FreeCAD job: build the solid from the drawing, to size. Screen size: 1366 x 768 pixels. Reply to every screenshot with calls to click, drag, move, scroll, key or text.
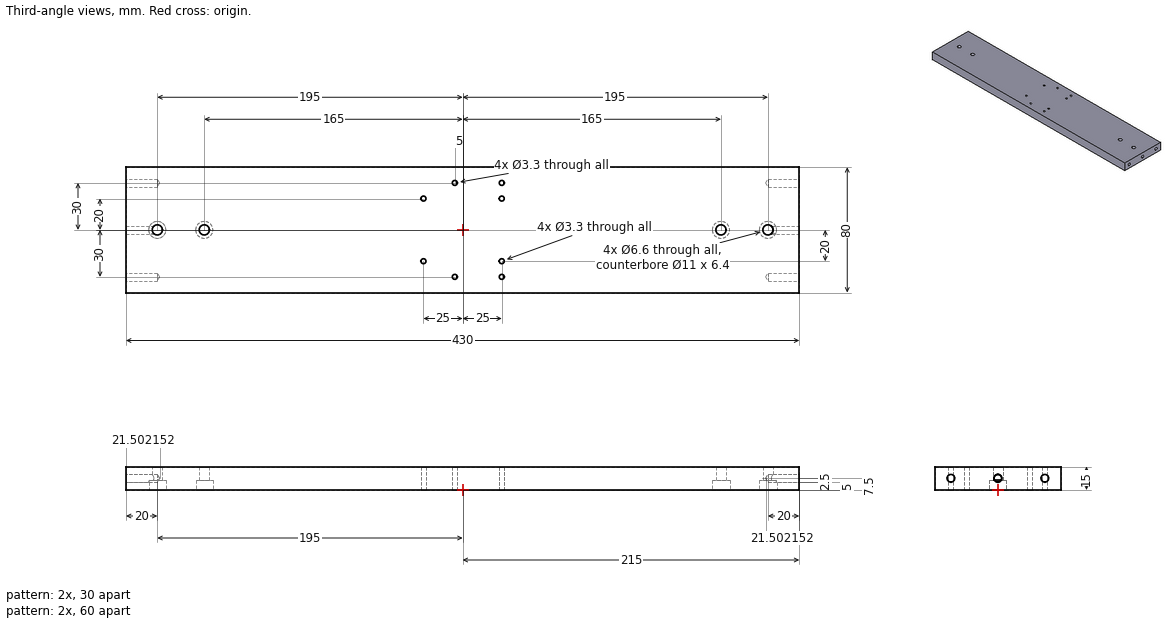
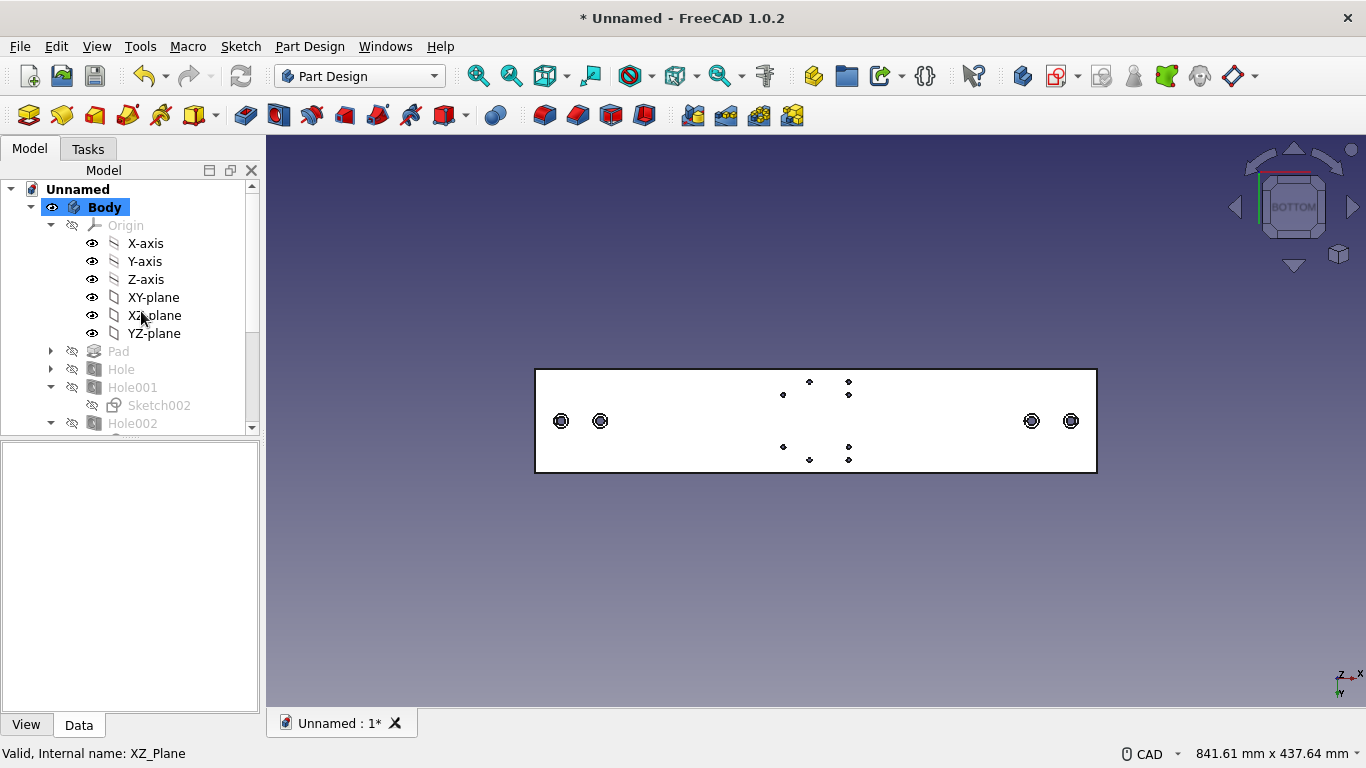
click(137, 315)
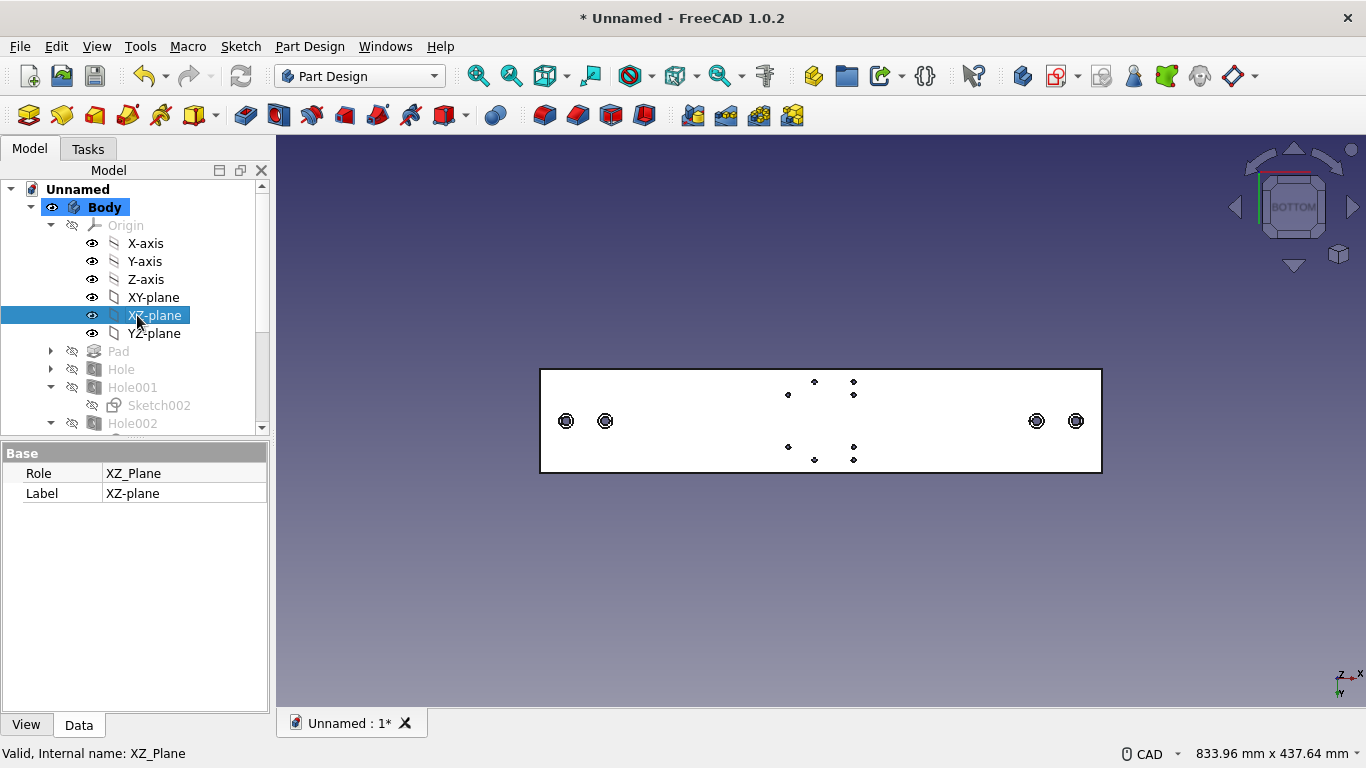
click(1232, 76)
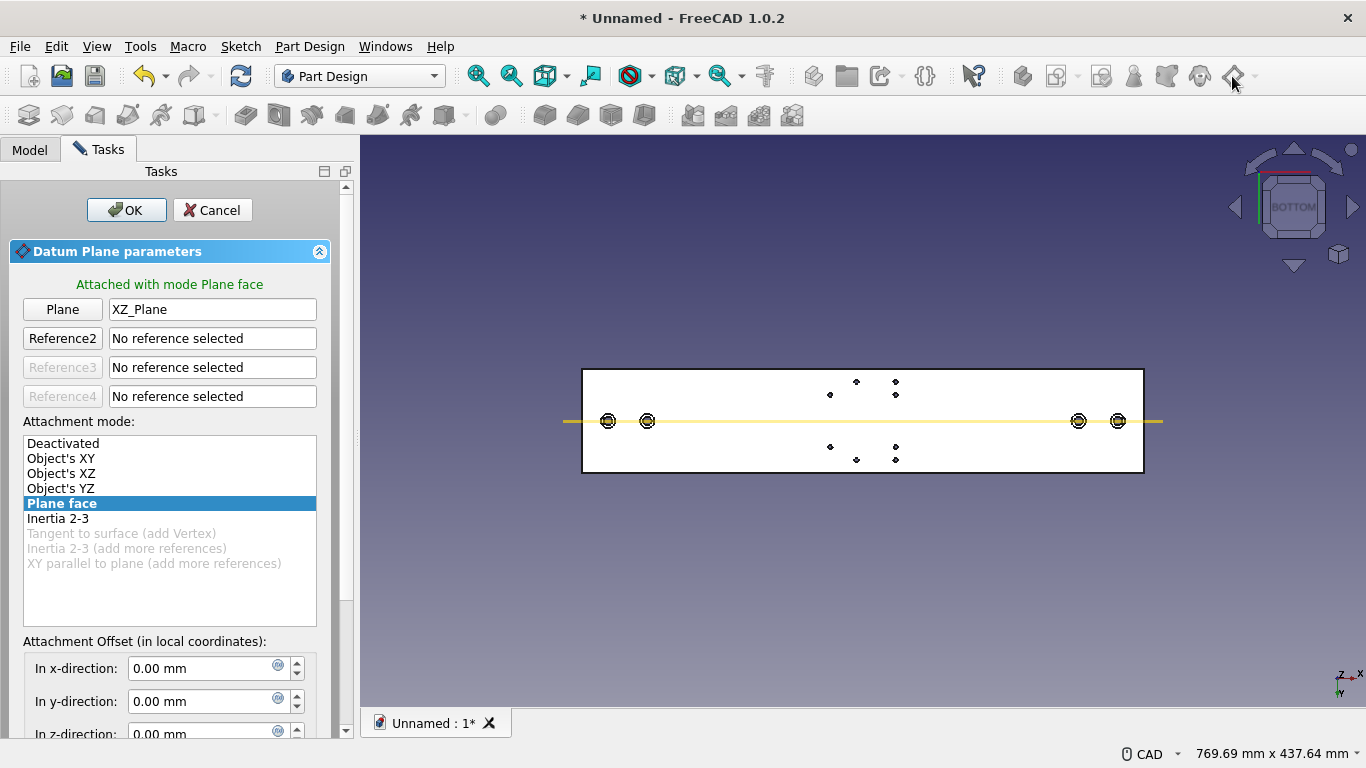
scroll(346, 460, down, 2)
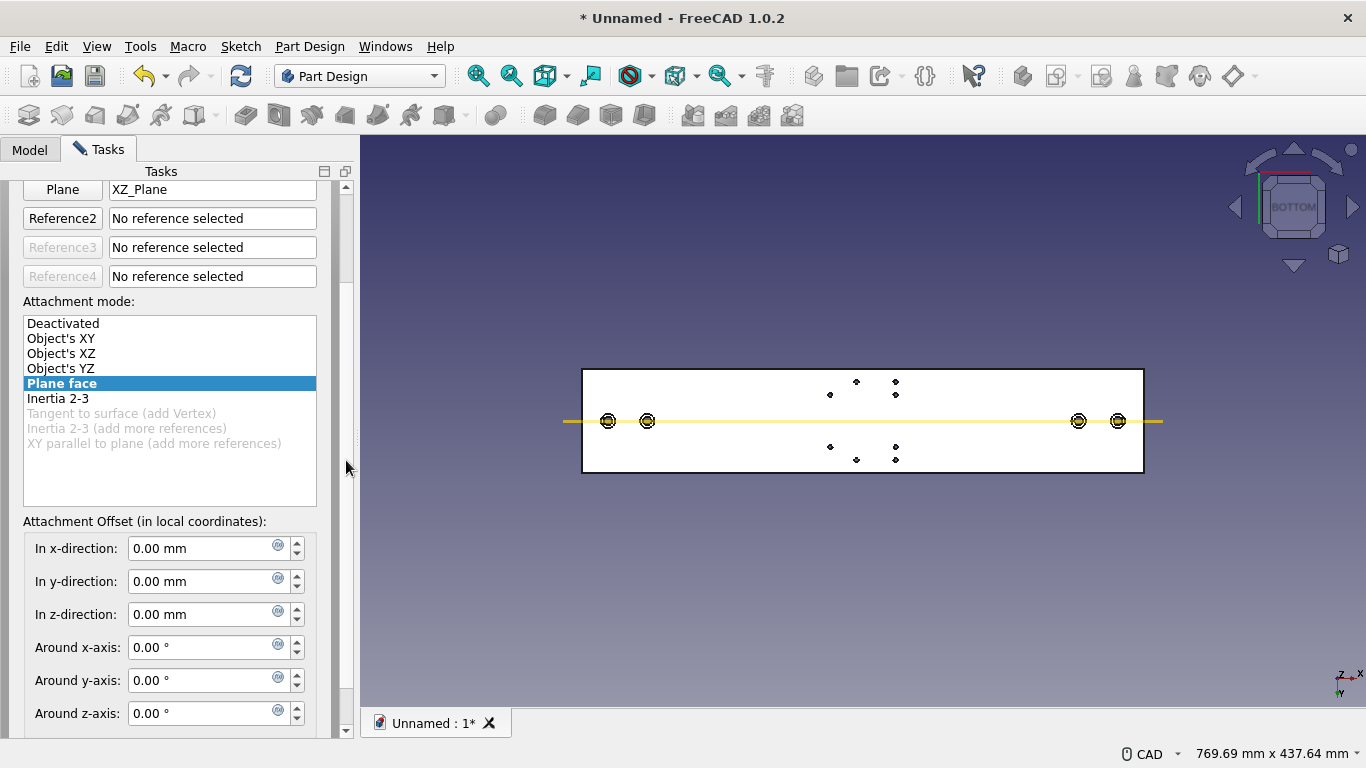
triple_click(210, 614)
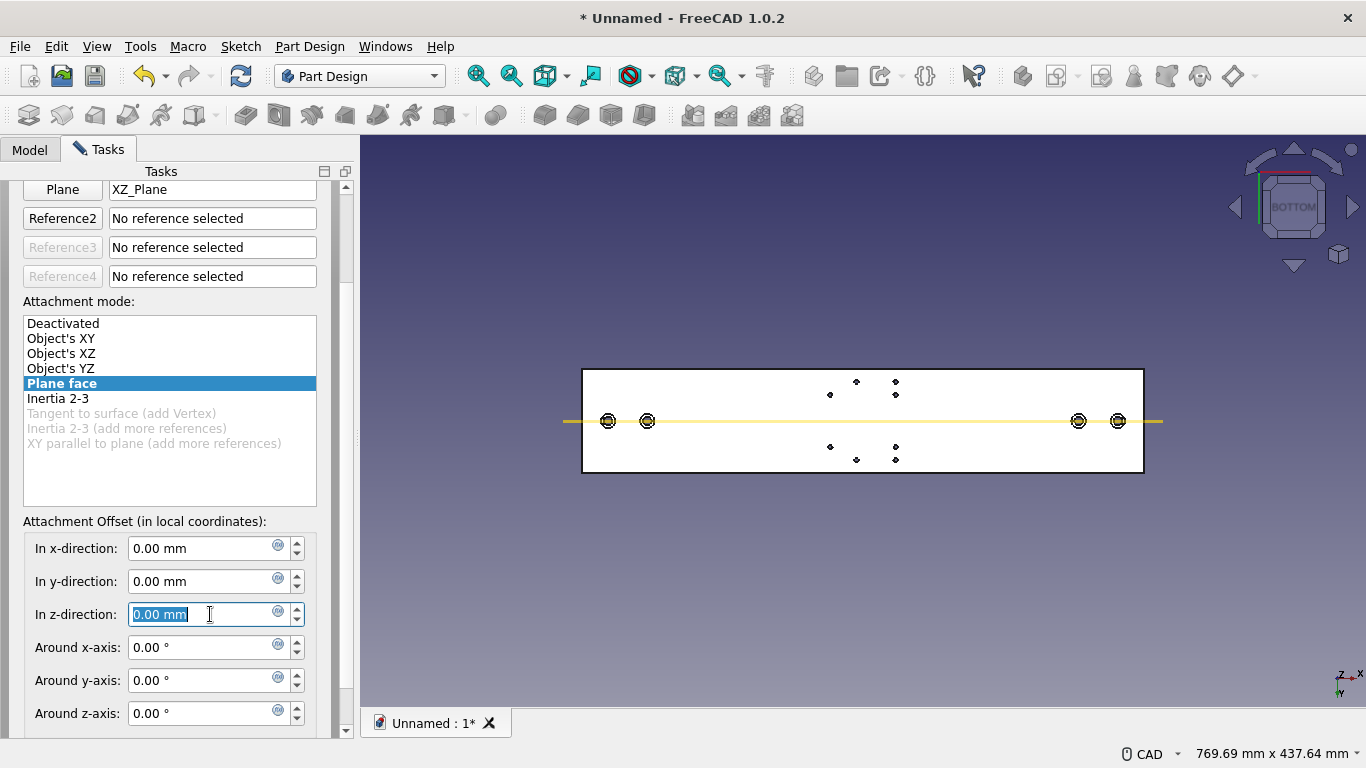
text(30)
key(Tab)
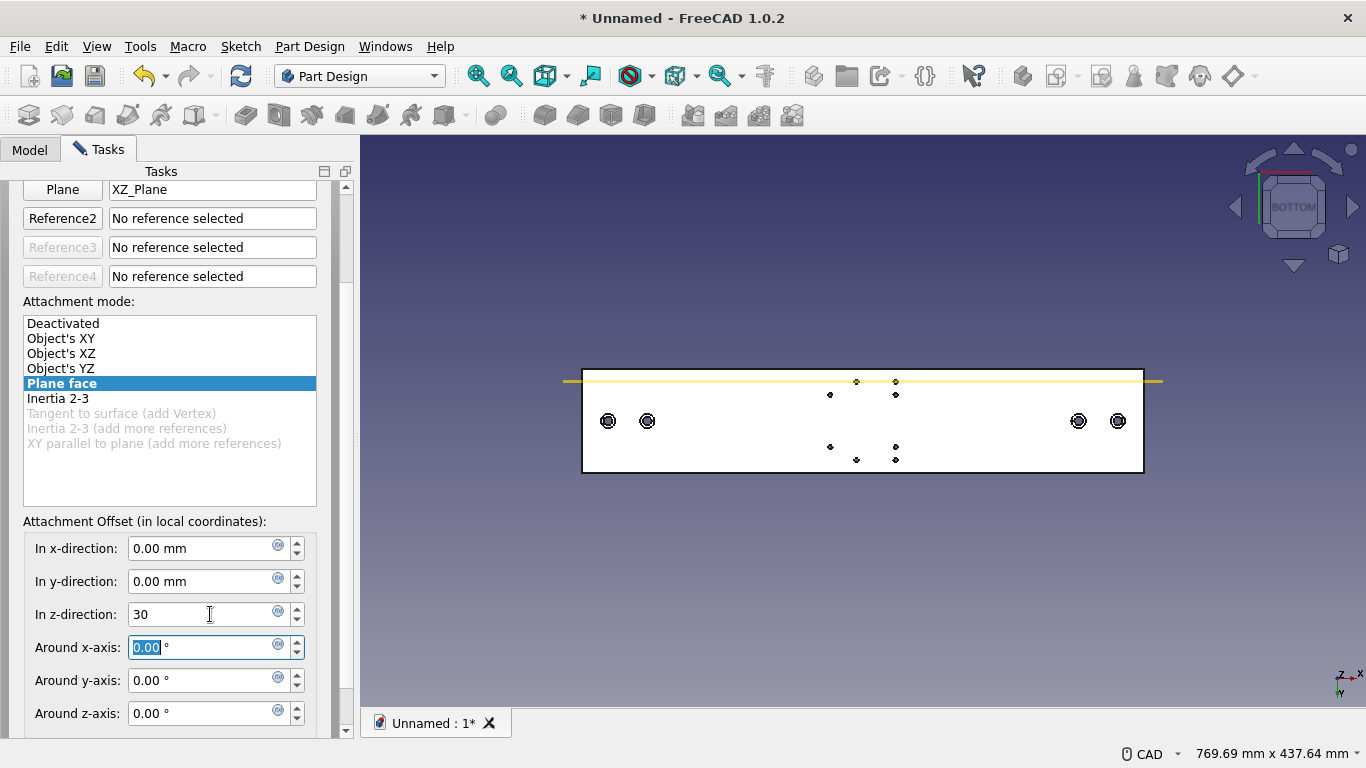
scroll(346, 460, up, 3)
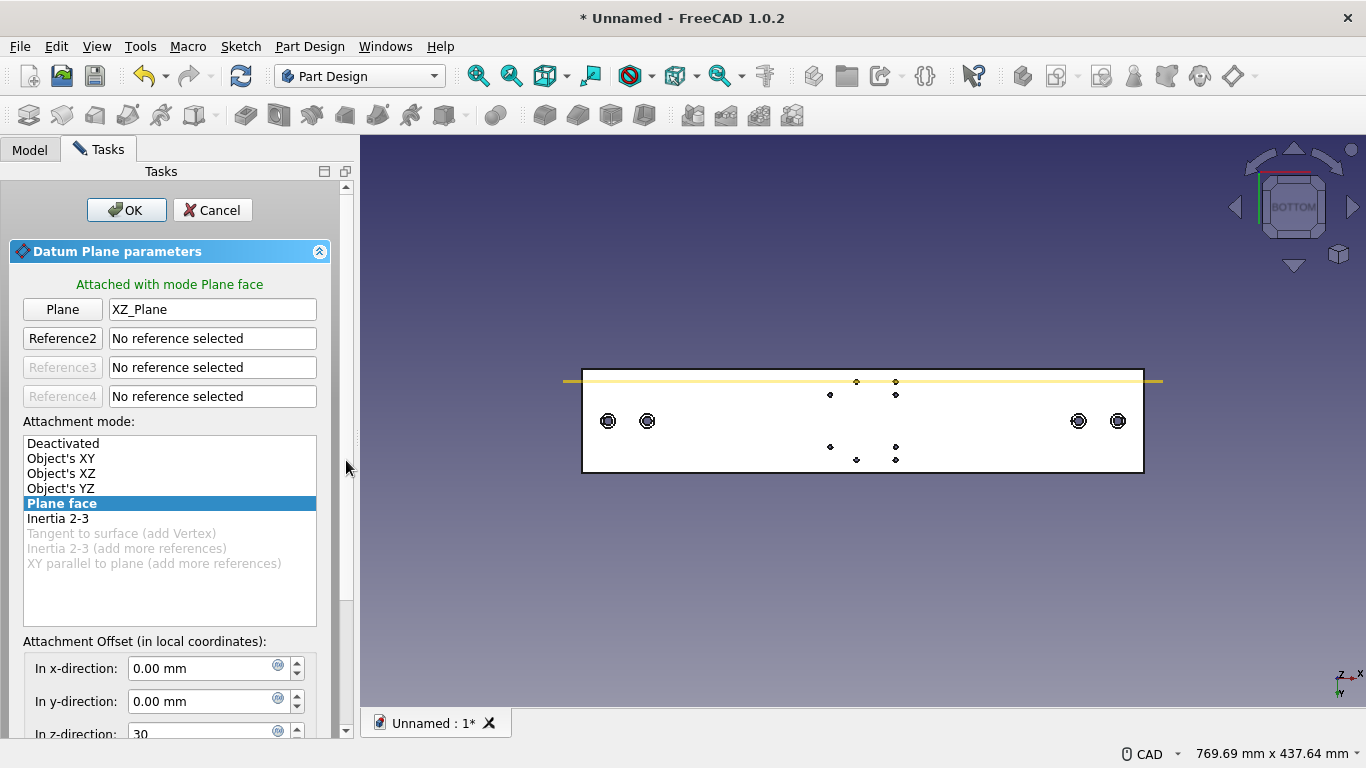
click(127, 210)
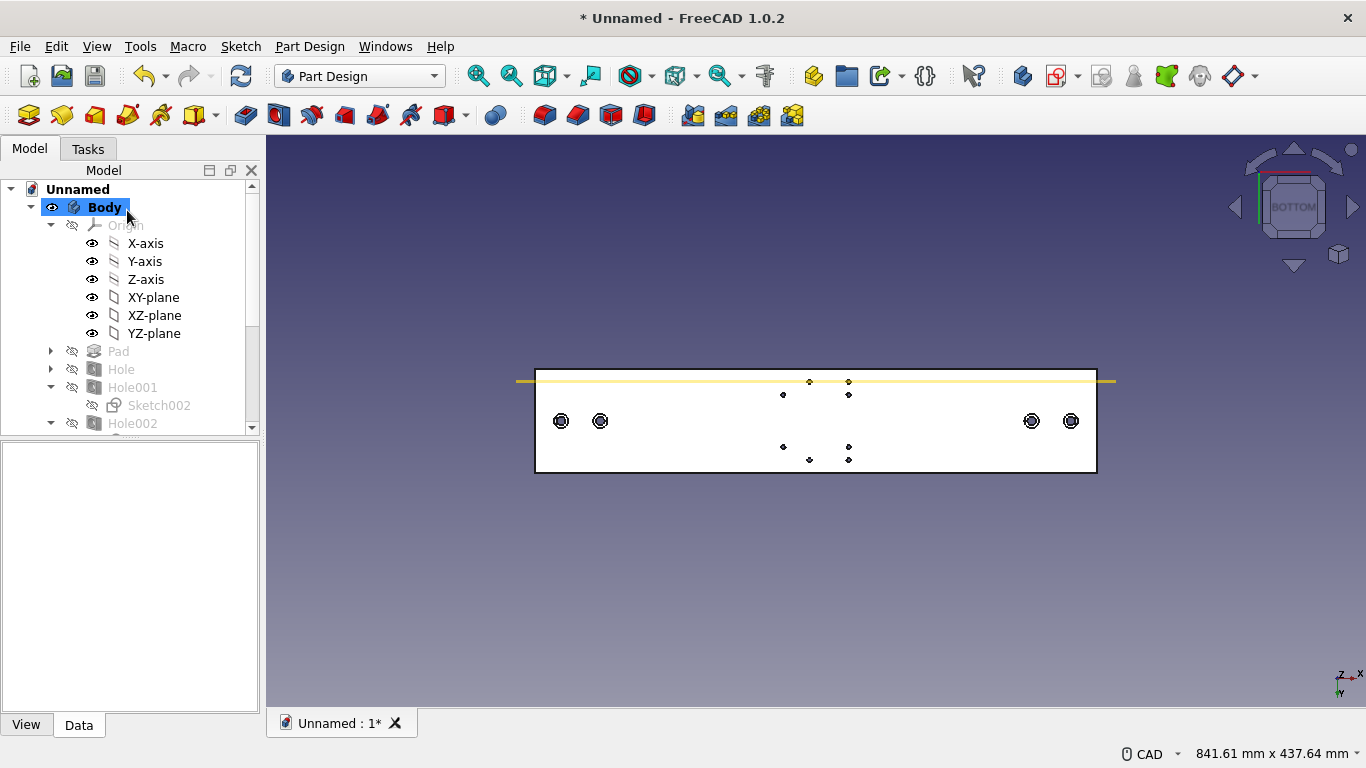
scroll(101, 311, down, 3)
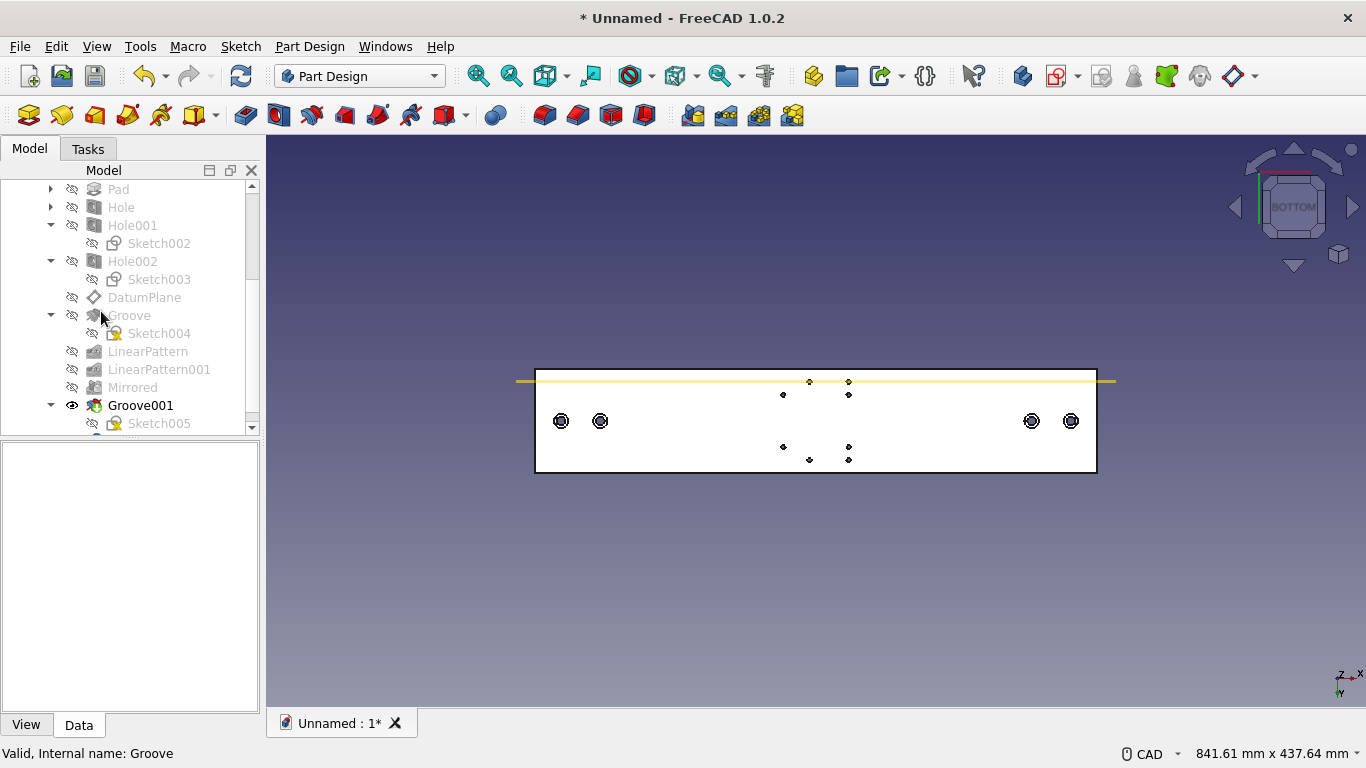
scroll(141, 311, up, 15)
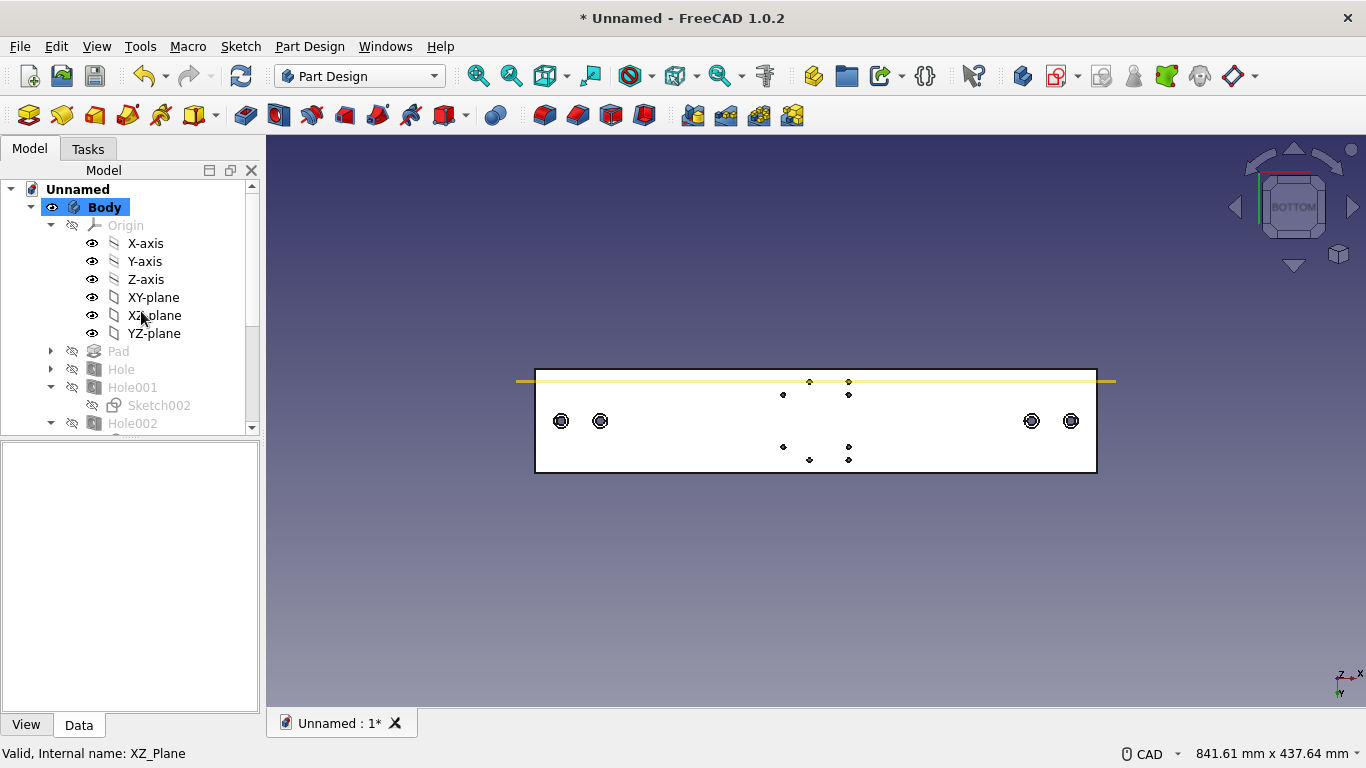
scroll(101, 311, down, 6)